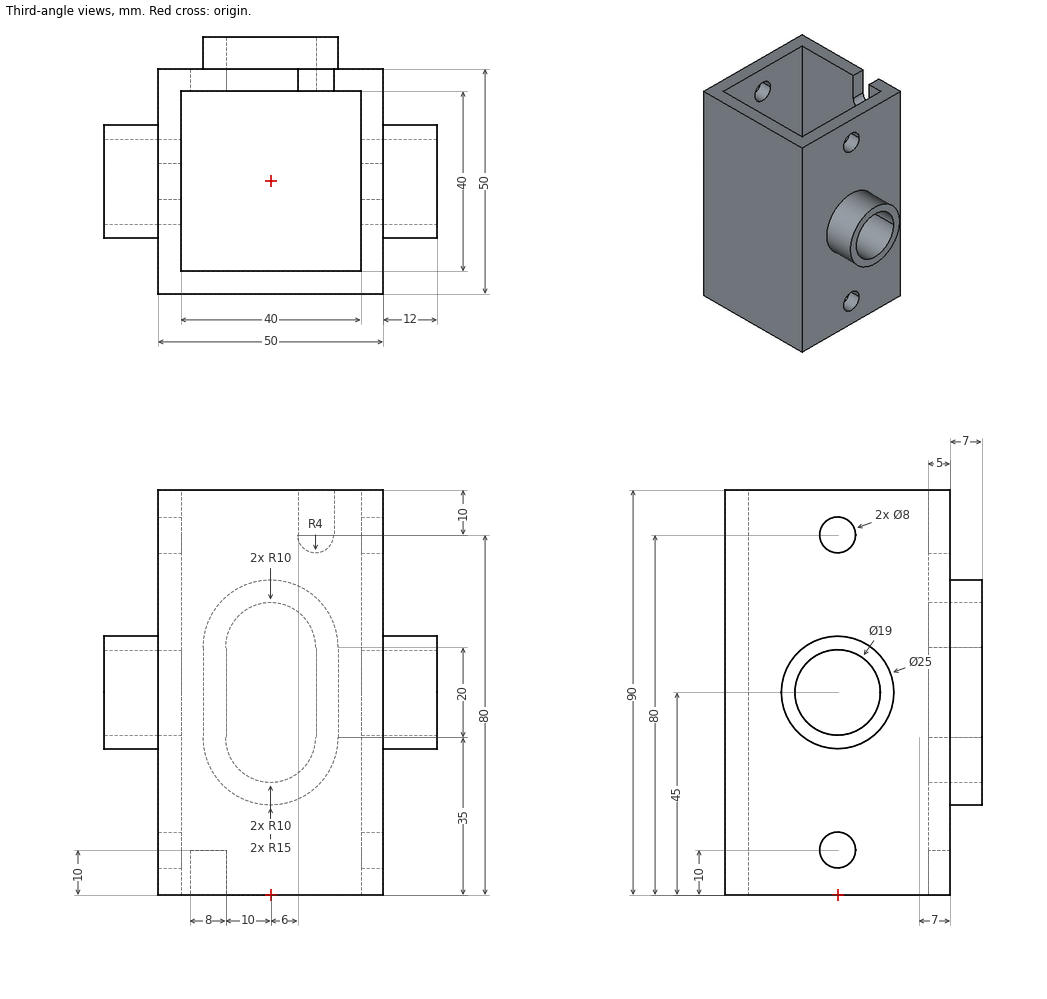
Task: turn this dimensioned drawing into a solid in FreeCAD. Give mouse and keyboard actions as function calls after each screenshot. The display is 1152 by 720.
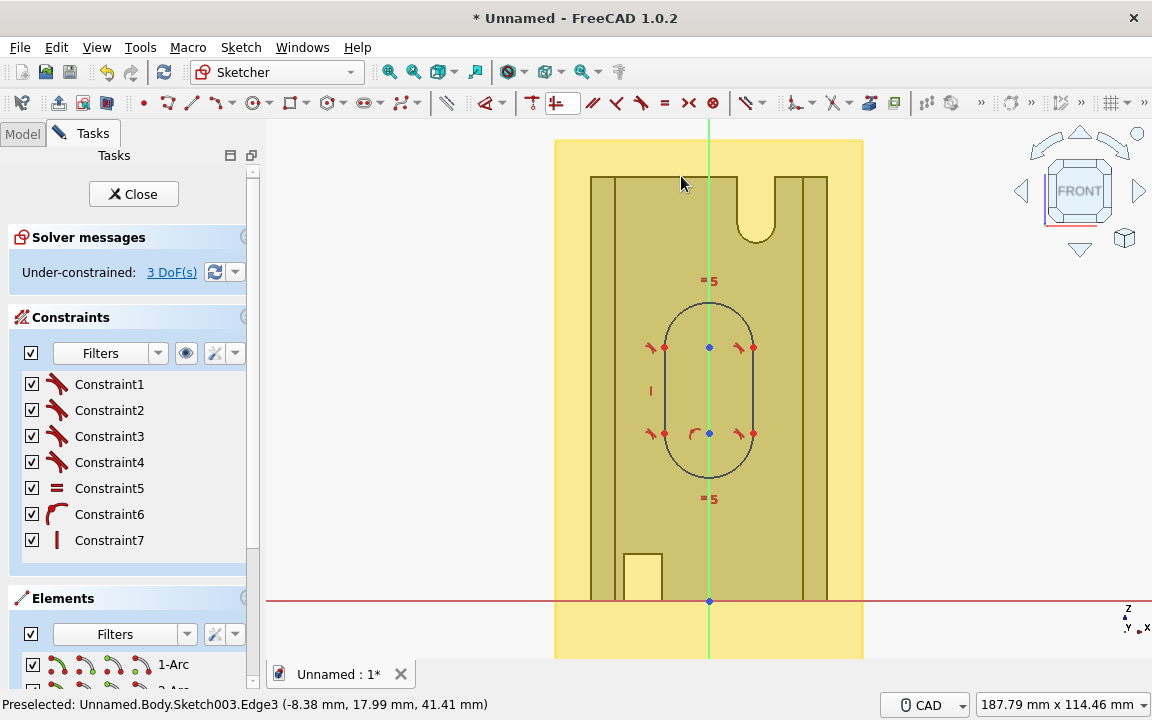
key(d)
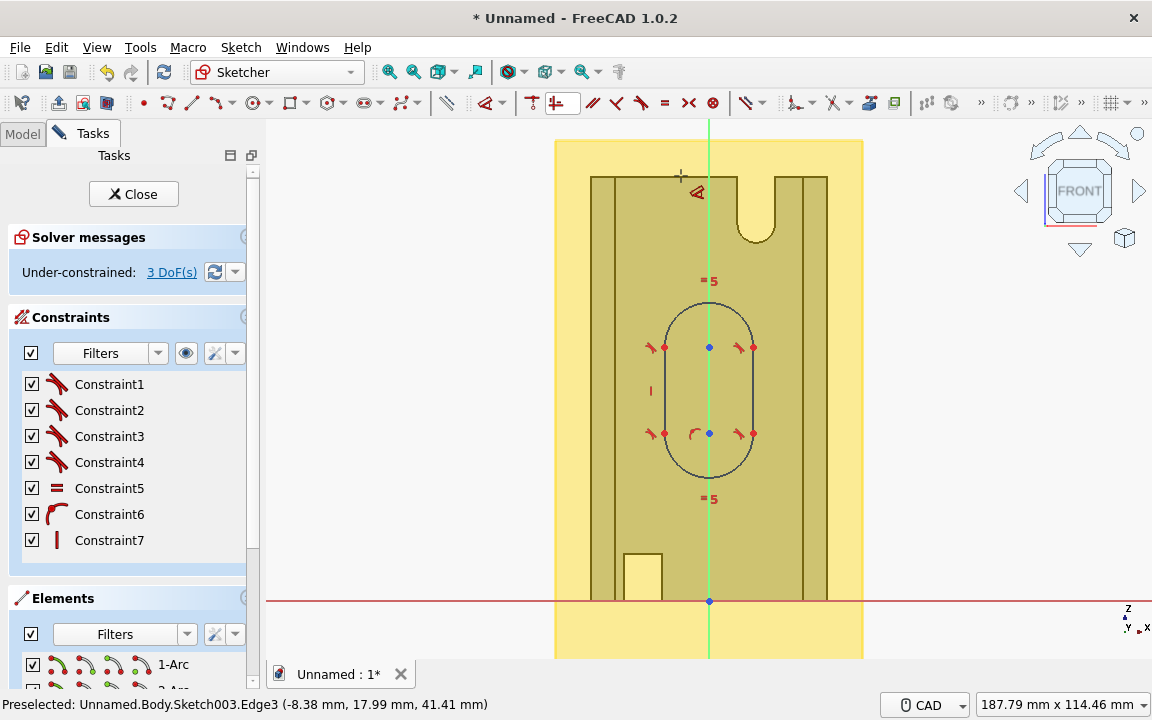
click(683, 469)
click(664, 495)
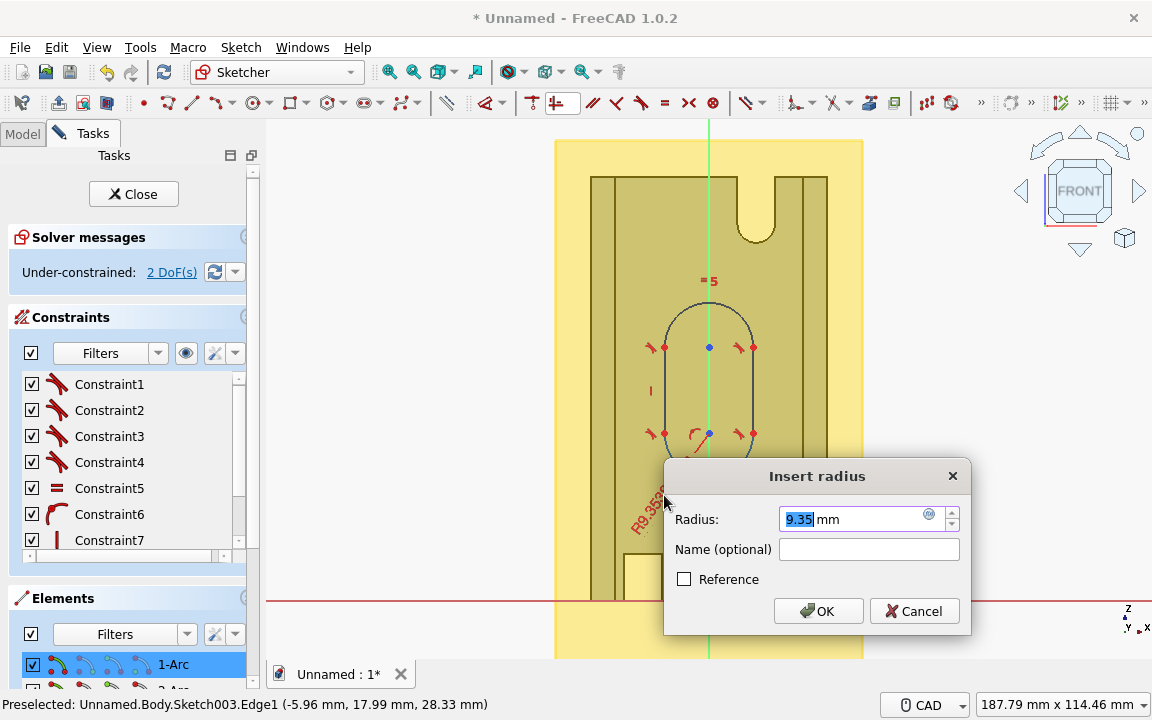
text(10)
key(Return)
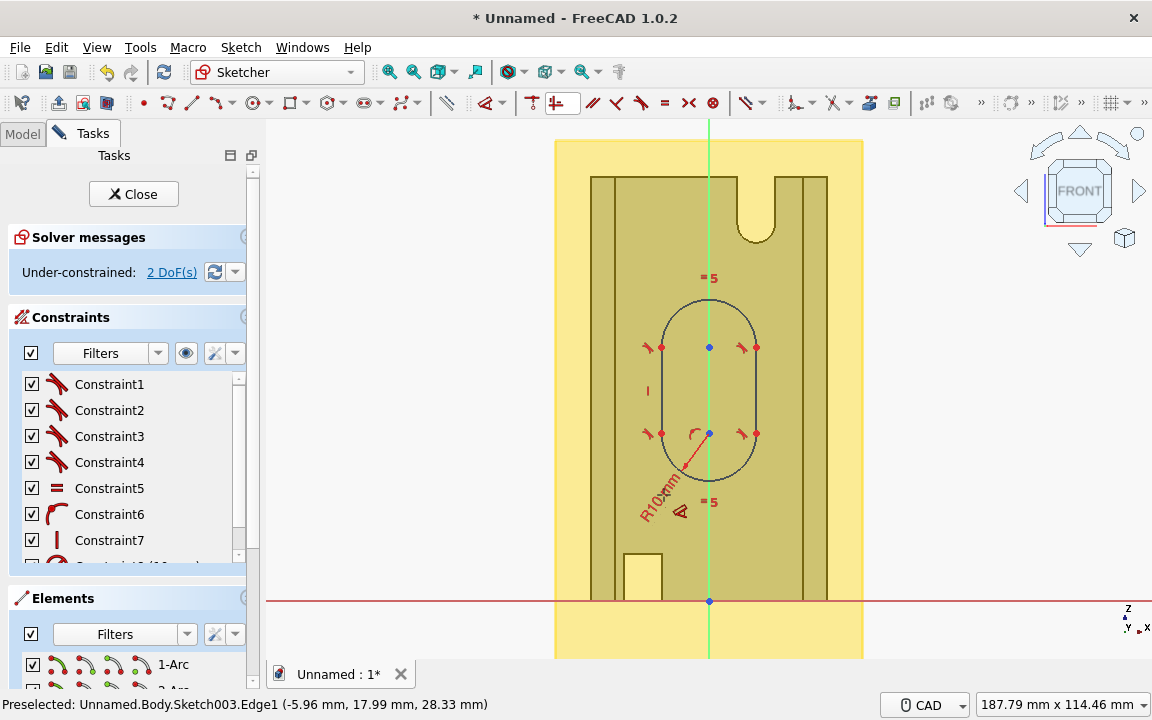
click(662, 408)
click(628, 390)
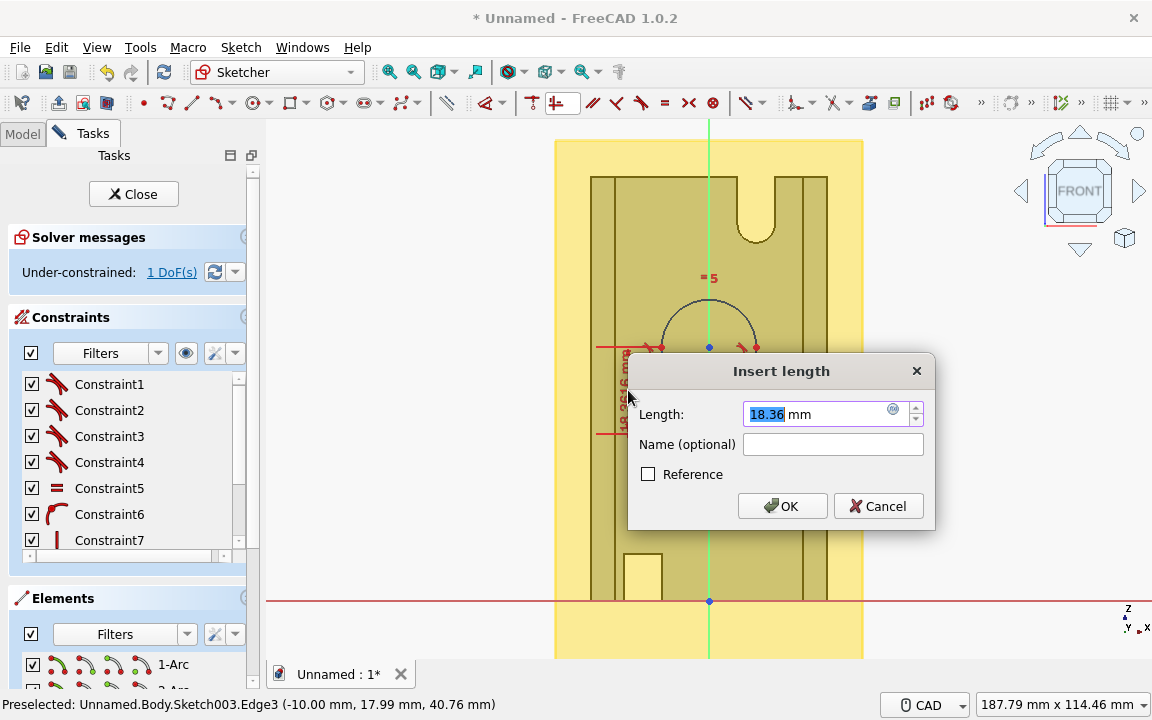
text(20)
key(Return)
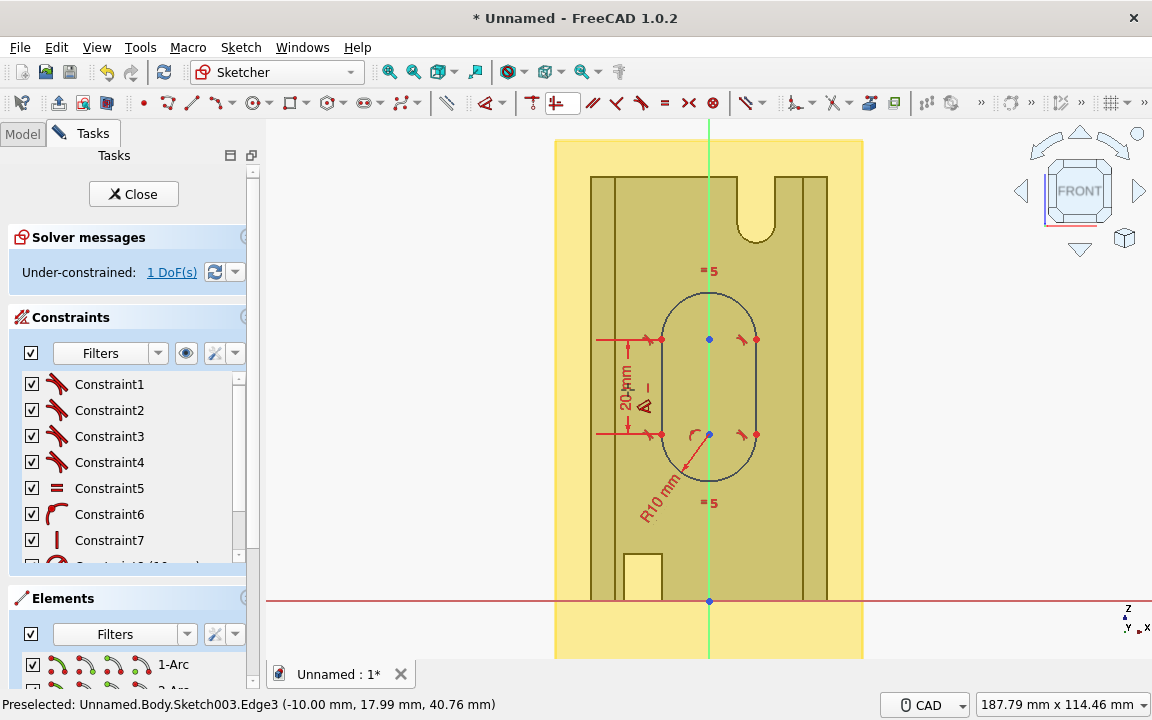
click(662, 434)
click(628, 518)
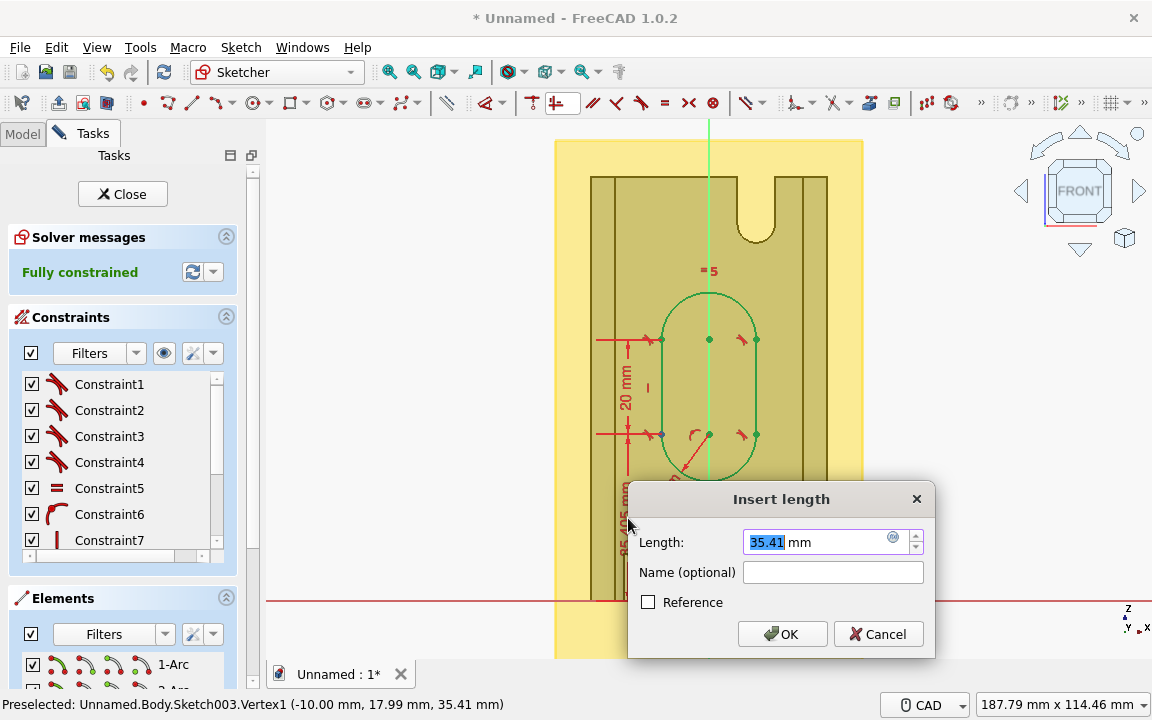
text(35)
key(Return)
key(Escape)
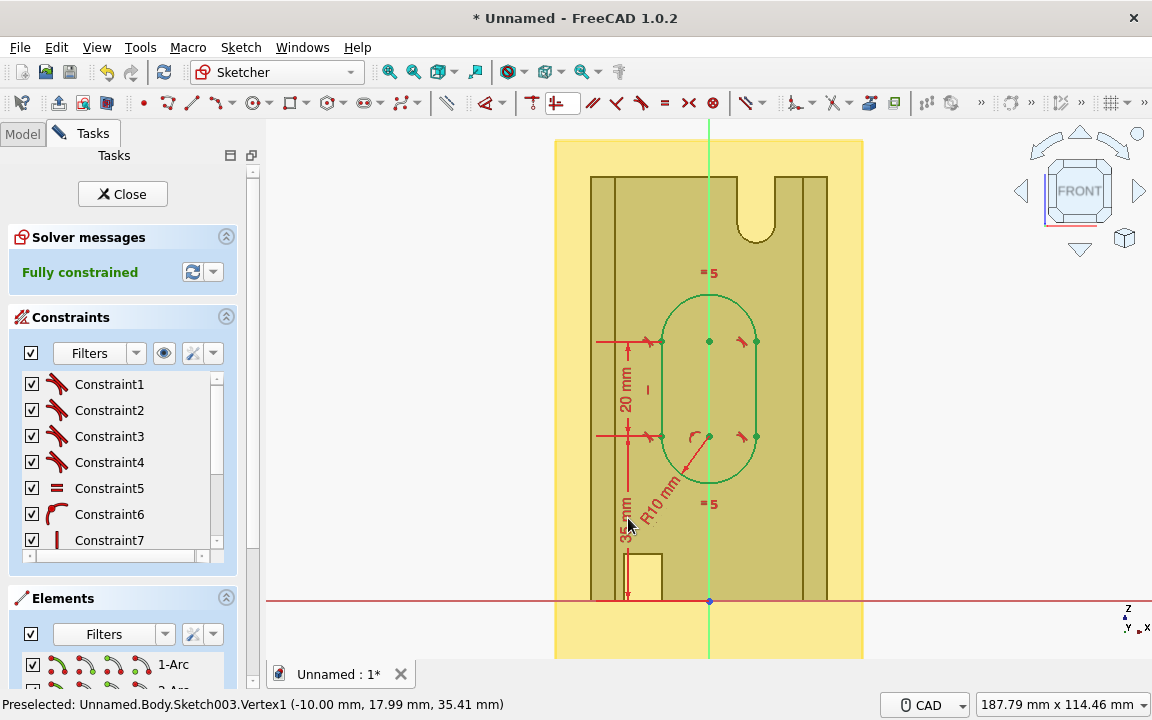
click(123, 194)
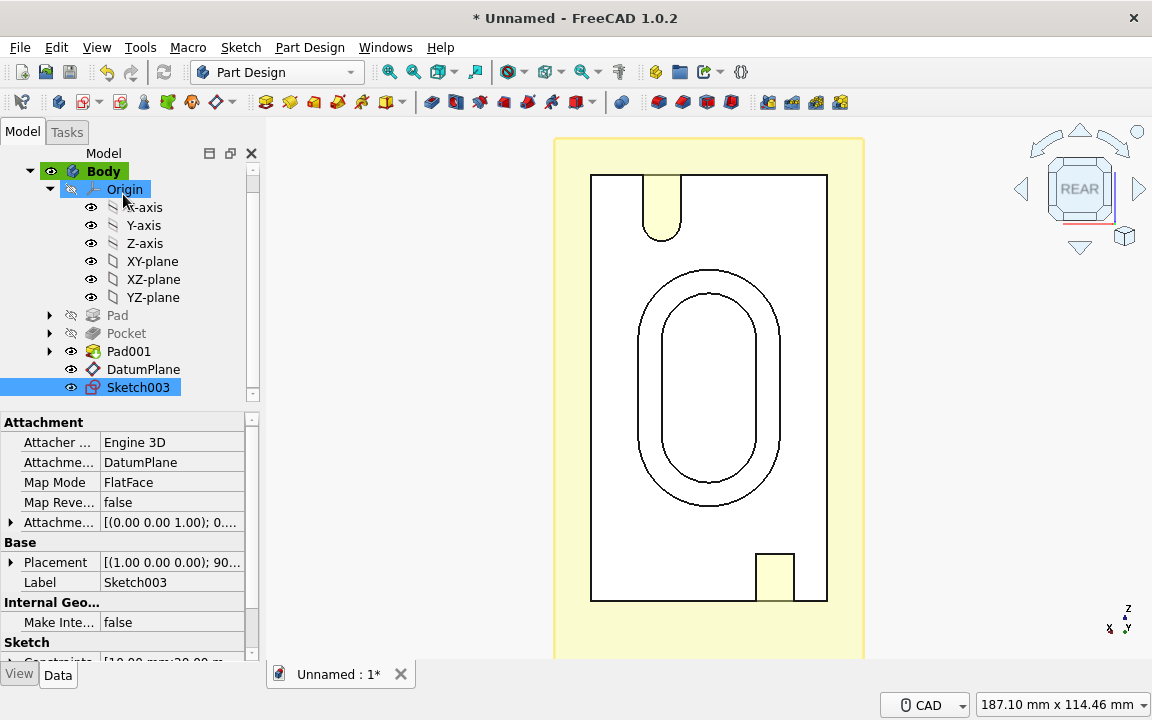
click(432, 102)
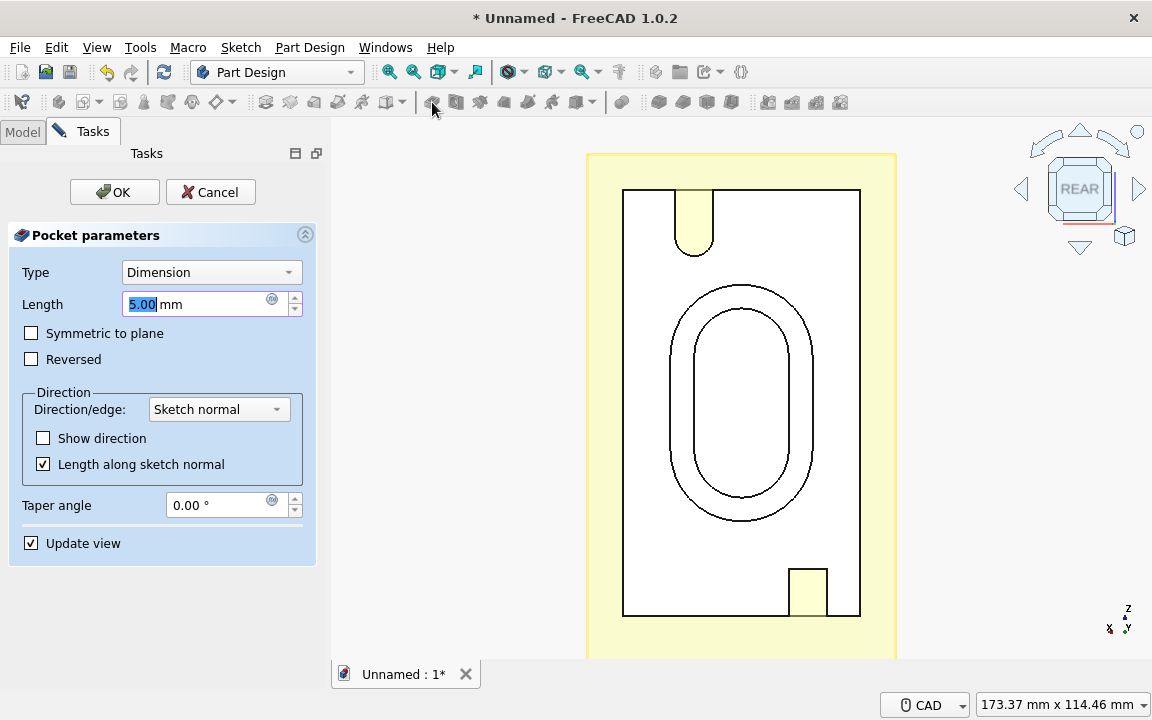
text(7)
key(Tab)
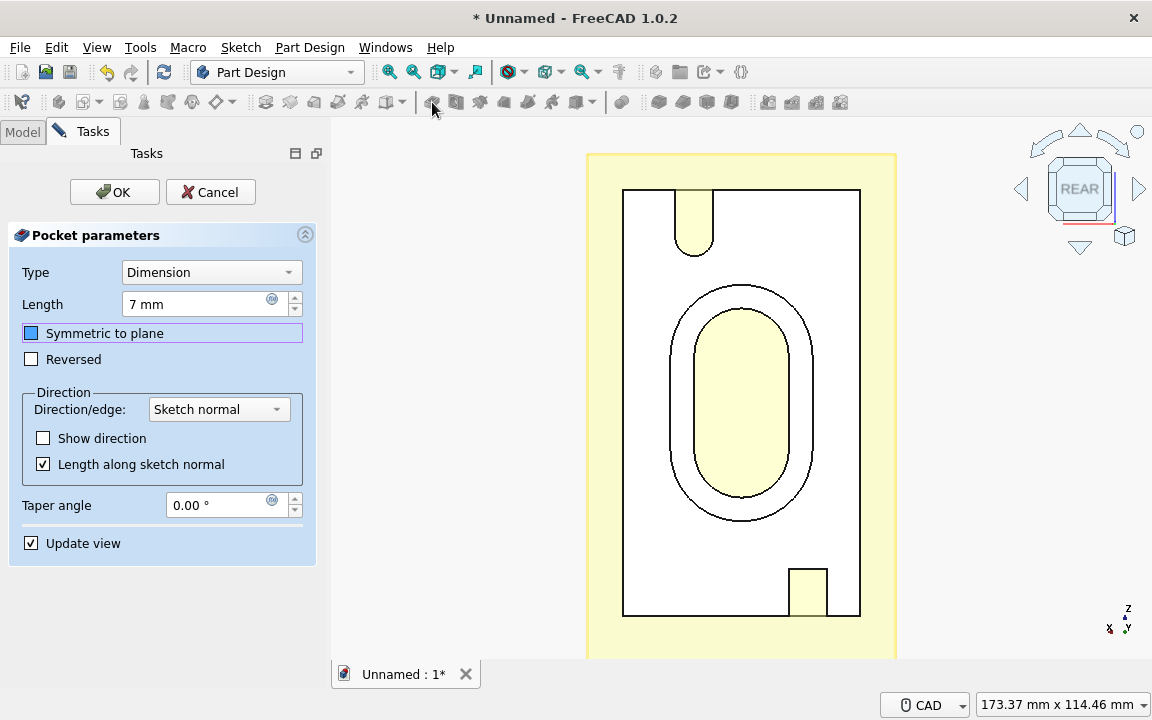
click(115, 192)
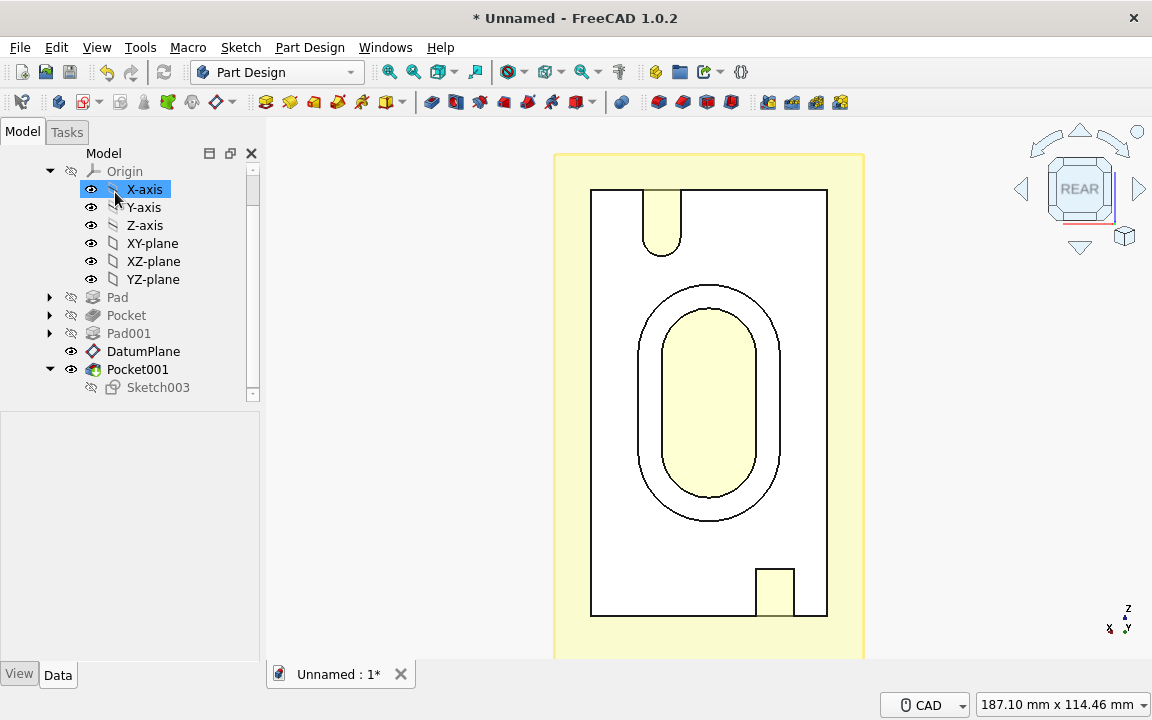
click(116, 351)
key(space)